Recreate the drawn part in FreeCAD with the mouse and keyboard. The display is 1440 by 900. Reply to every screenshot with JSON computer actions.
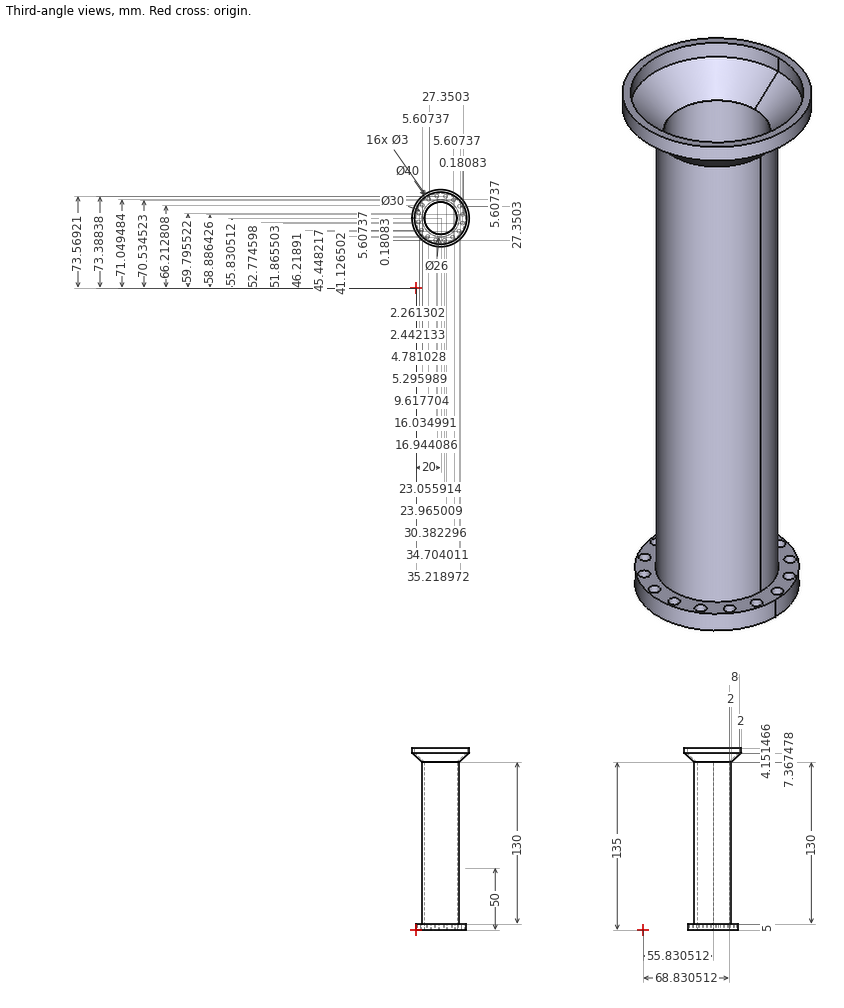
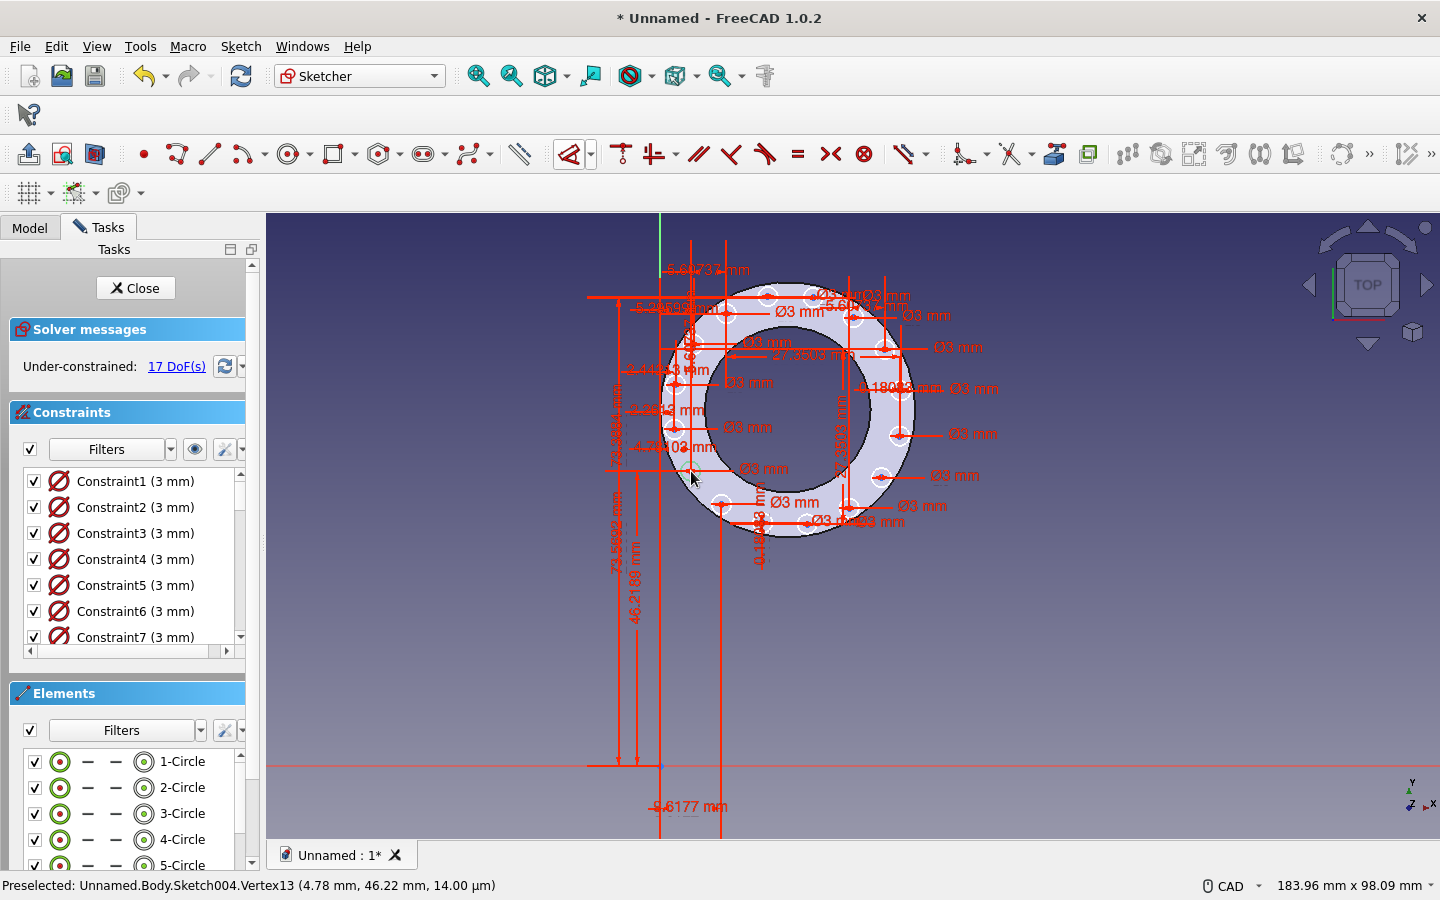
{"action": "left_click", "coordinate": [849, 508]}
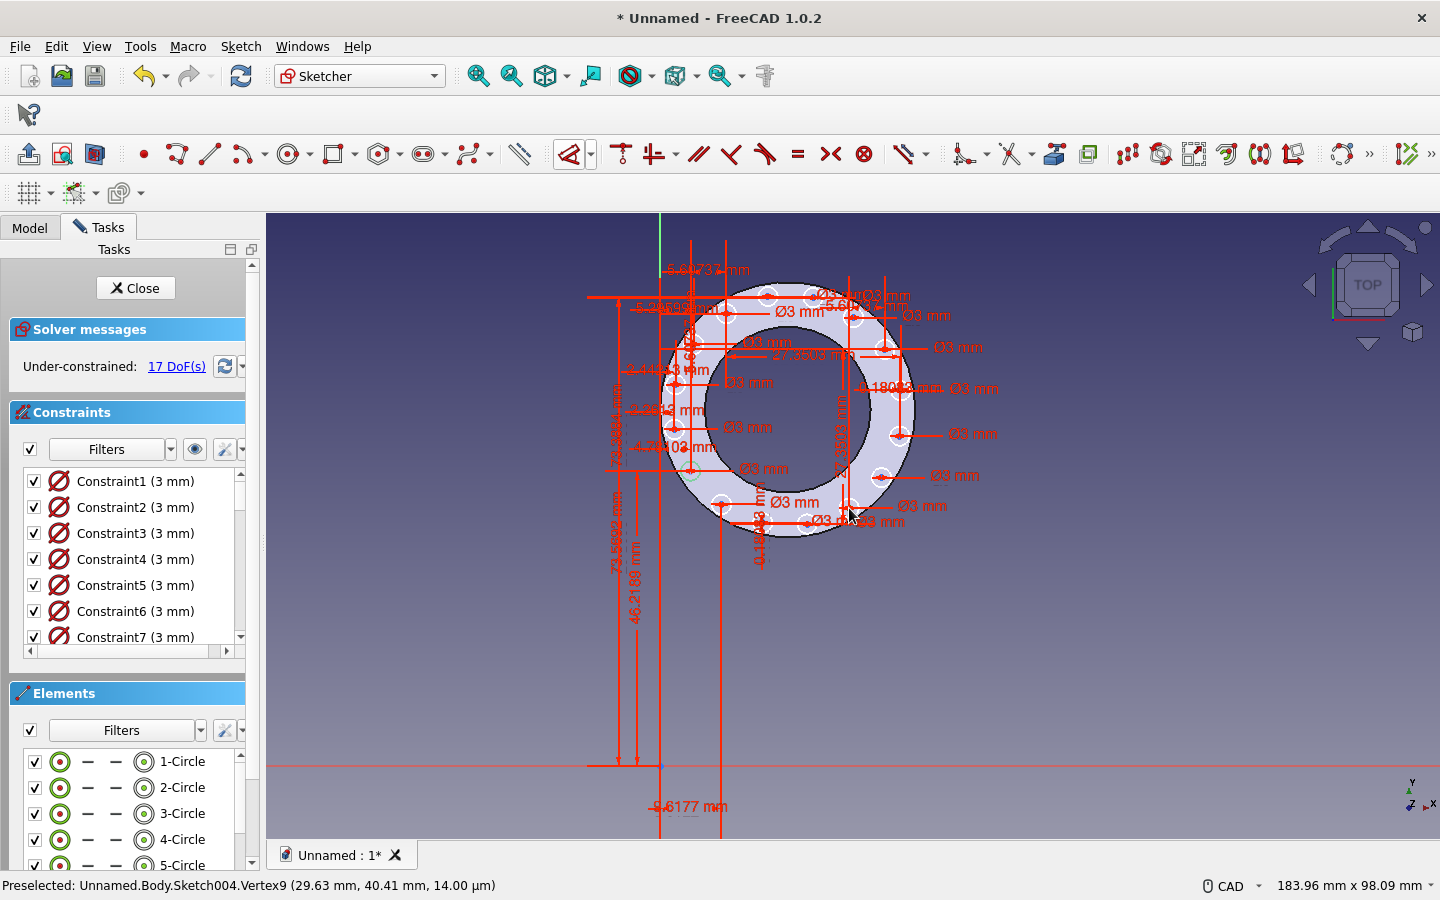
{"action": "left_click", "coordinate": [691, 471]}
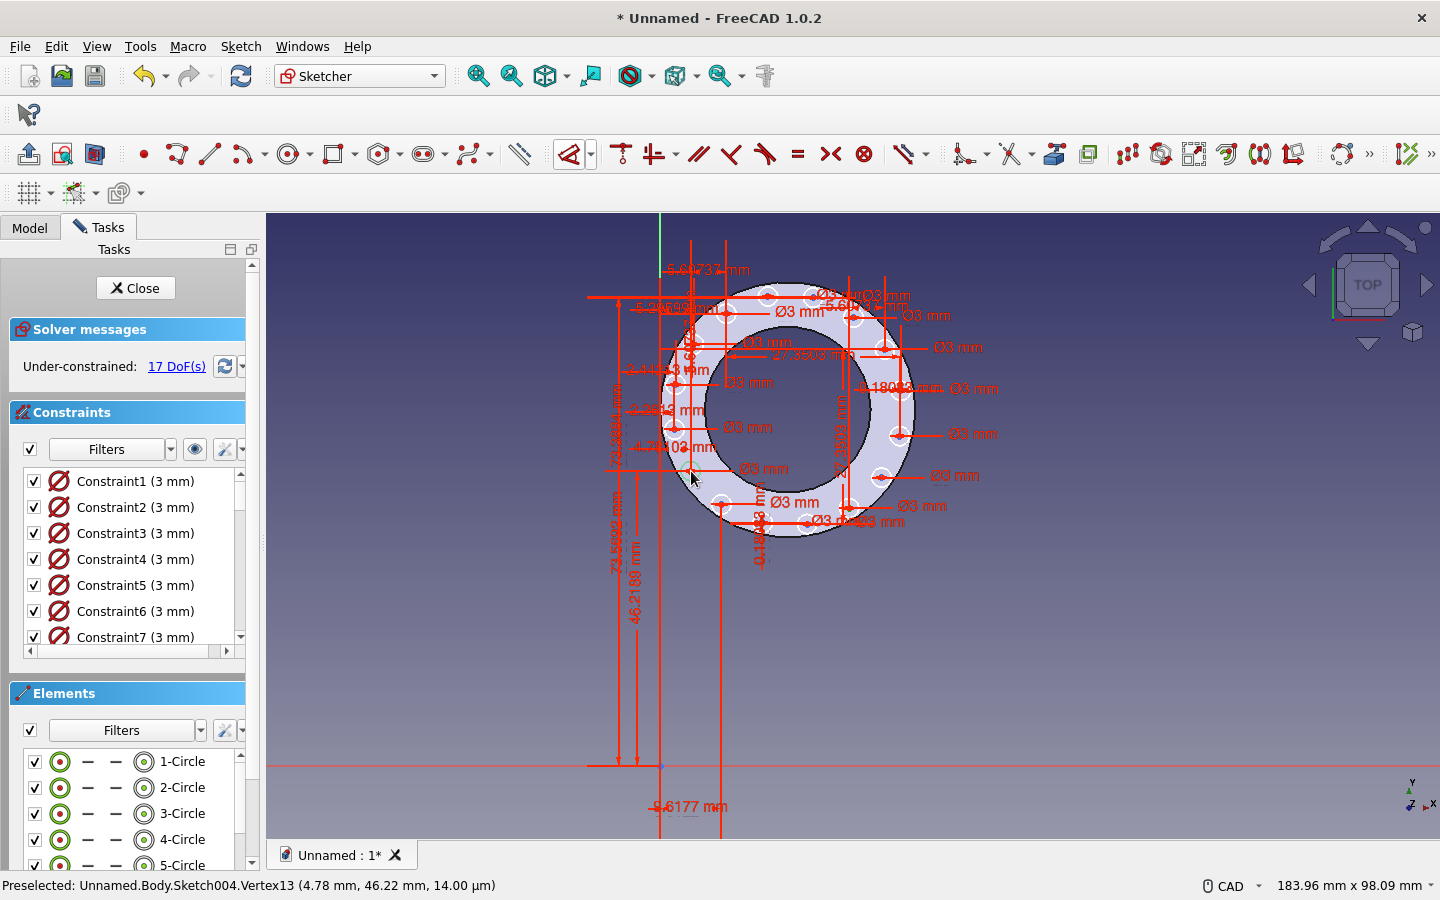
{"action": "key", "text": "i"}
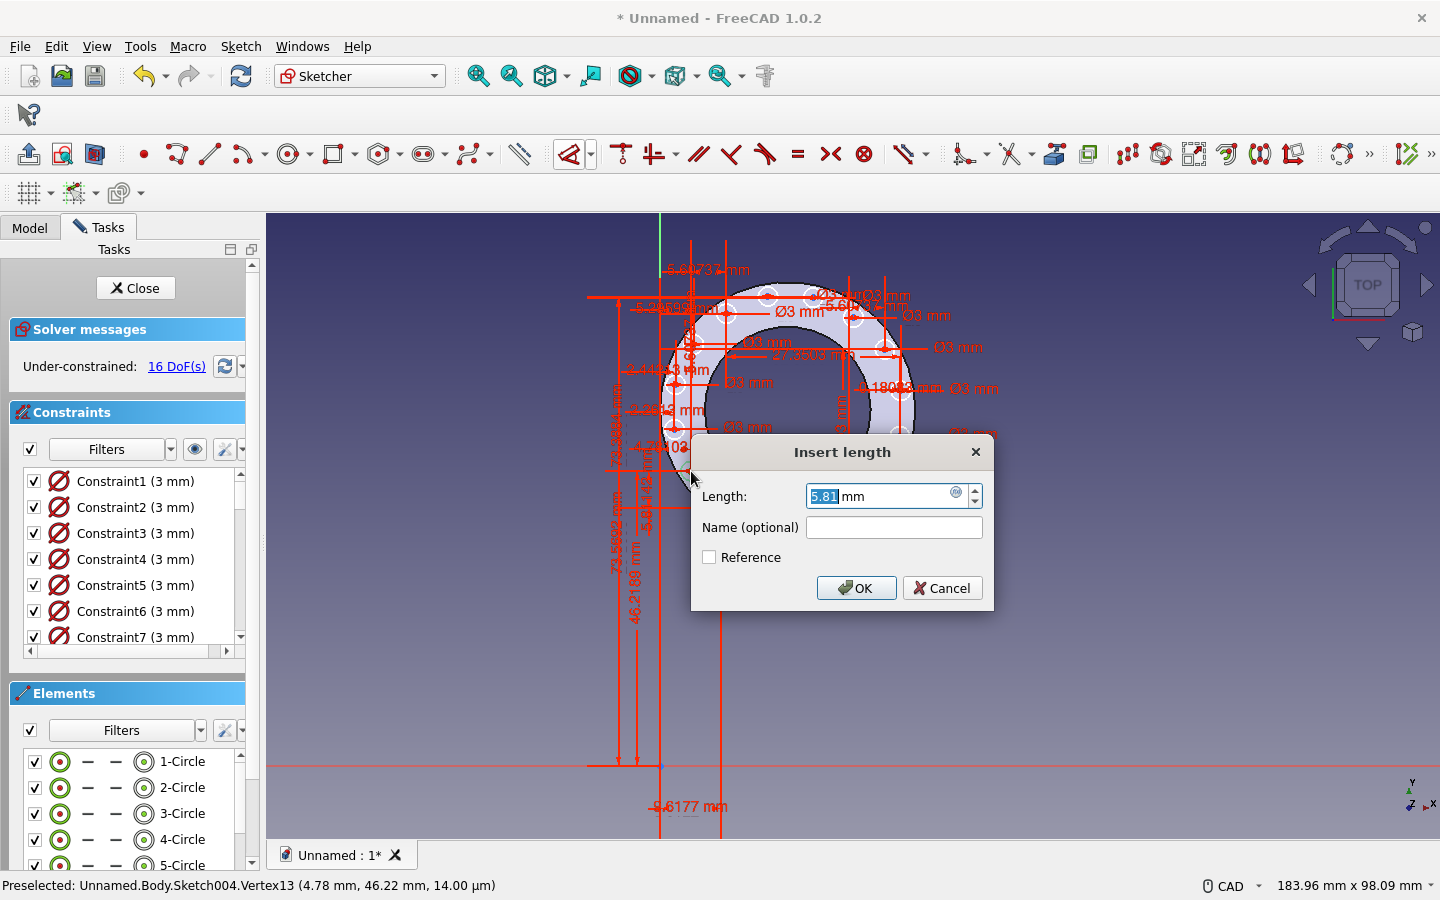
{"action": "type", "text": "5.60737"}
{"action": "key", "text": "Return"}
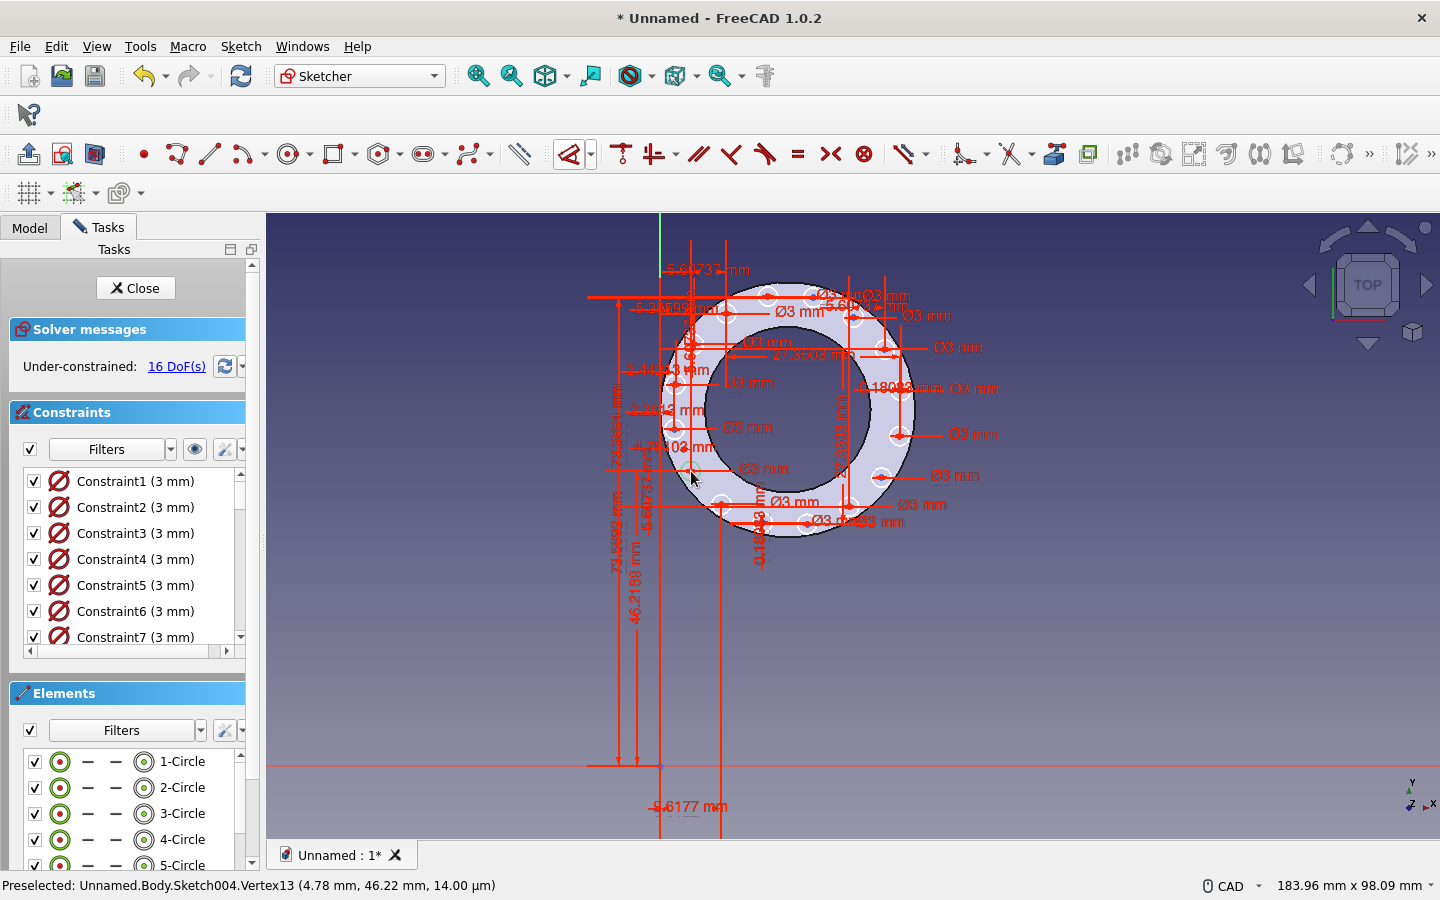
{"action": "left_click", "coordinate": [726, 314]}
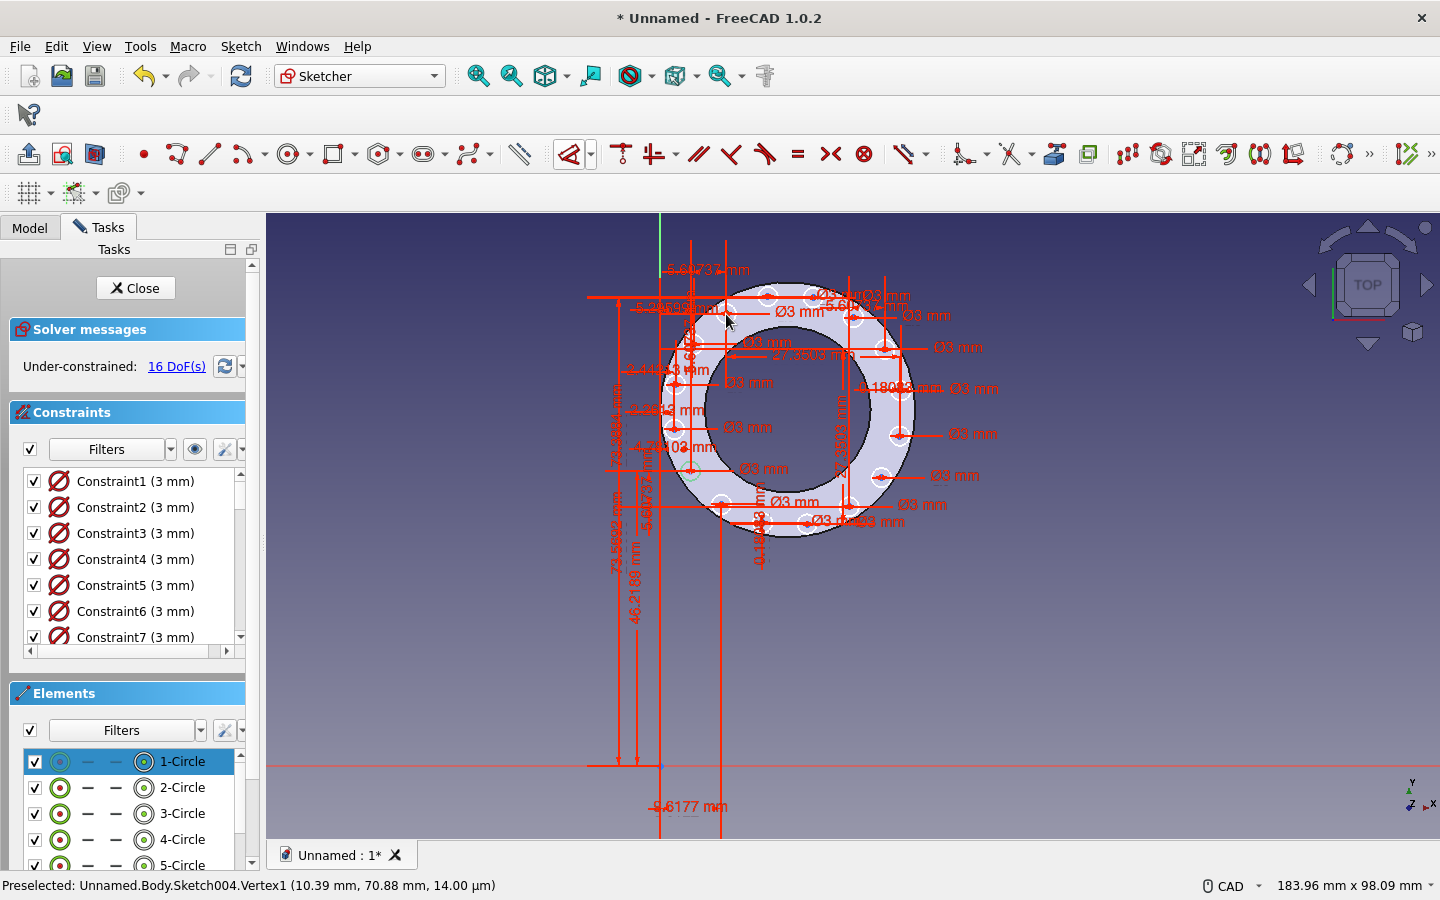
{"action": "left_click", "coordinate": [590, 154]}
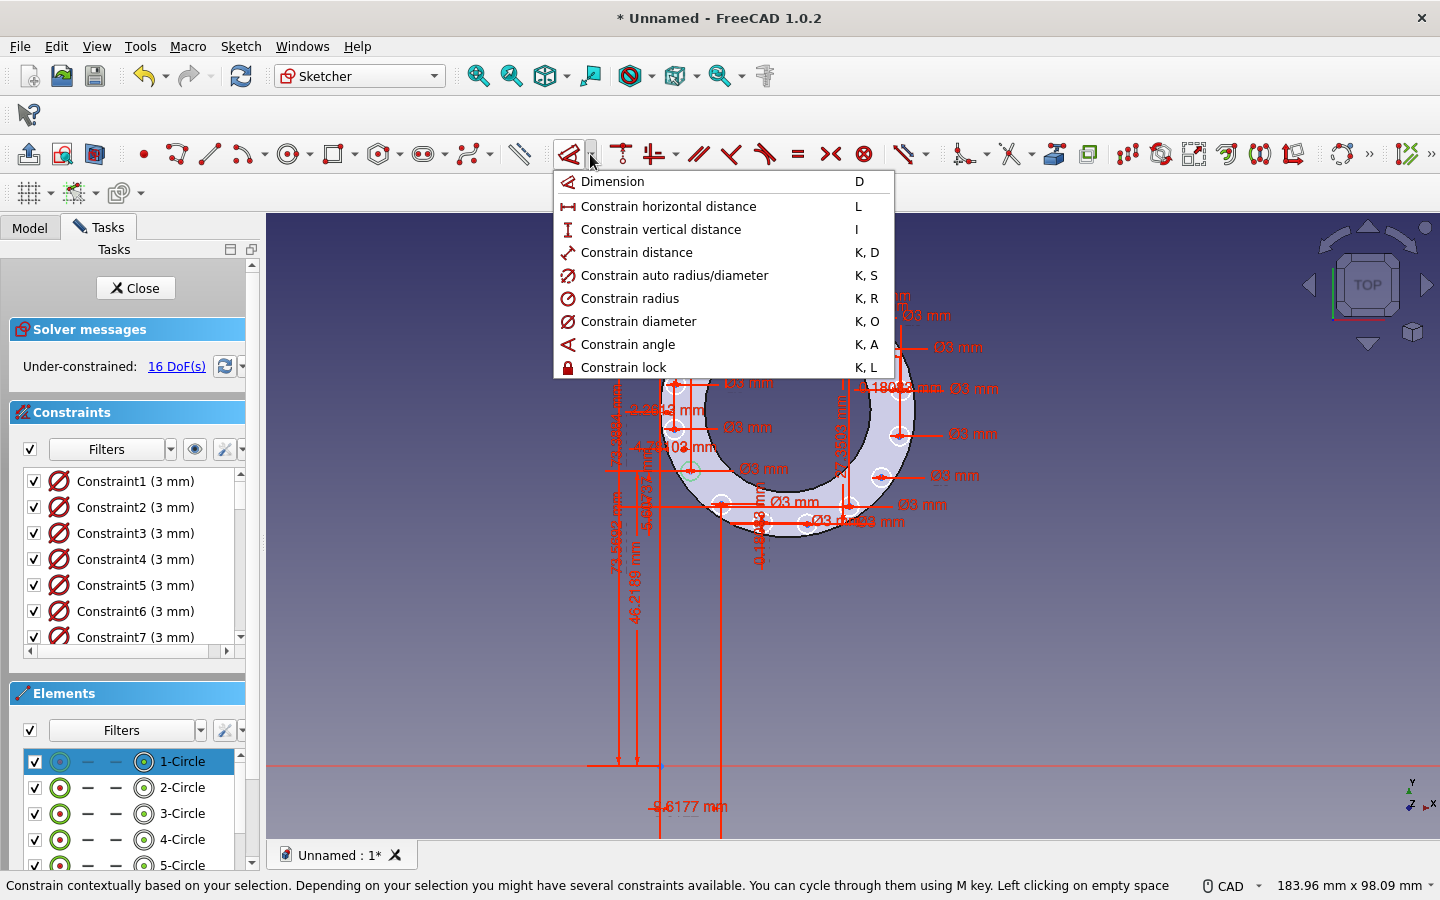
{"action": "left_click", "coordinate": [724, 230]}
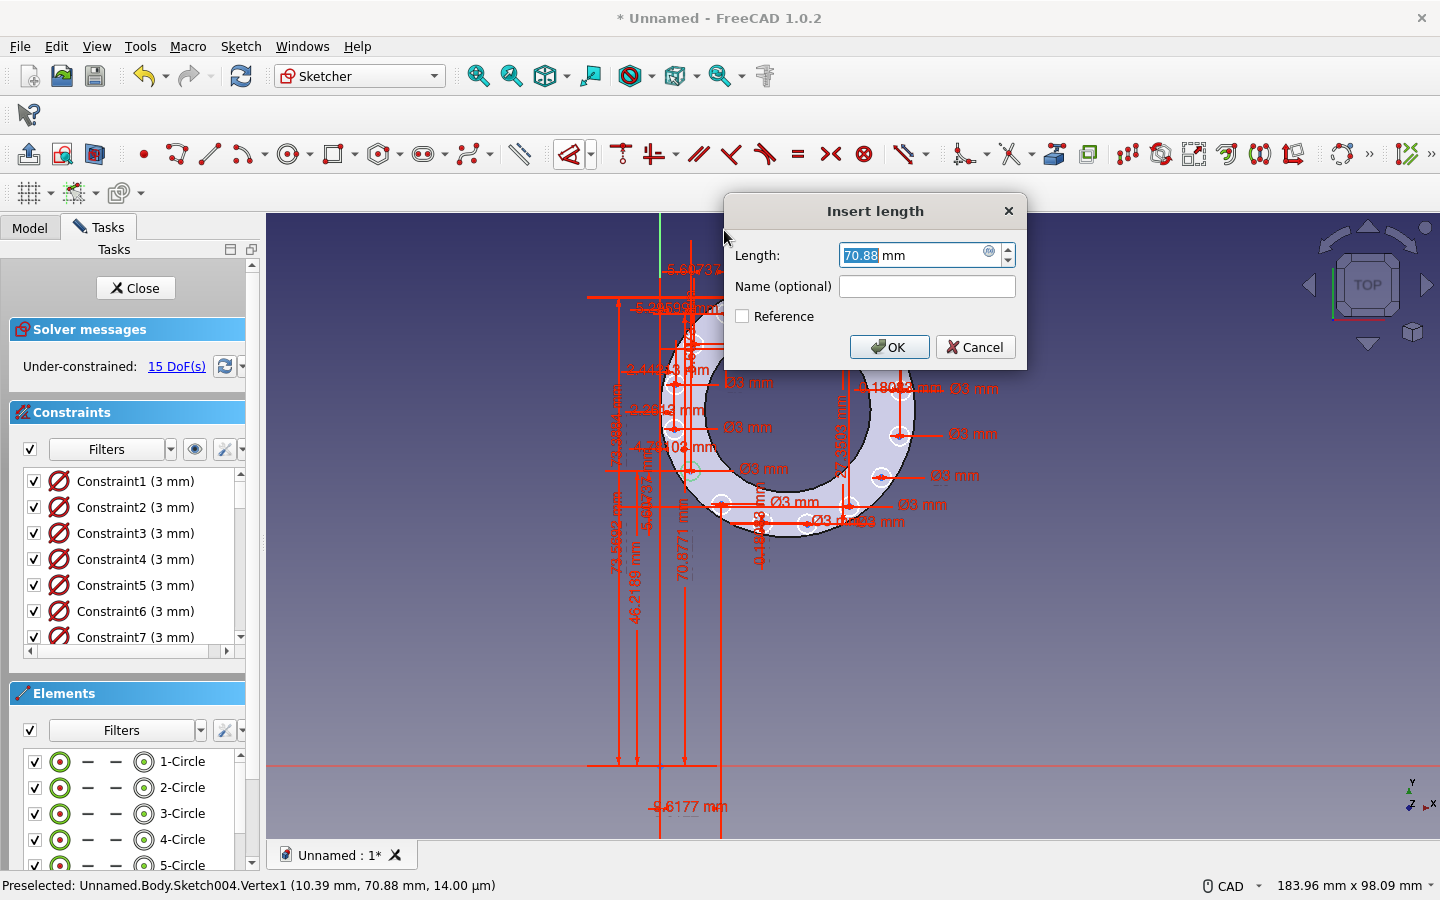
{"action": "type", "text": "71.049484"}
{"action": "key", "text": "Return"}